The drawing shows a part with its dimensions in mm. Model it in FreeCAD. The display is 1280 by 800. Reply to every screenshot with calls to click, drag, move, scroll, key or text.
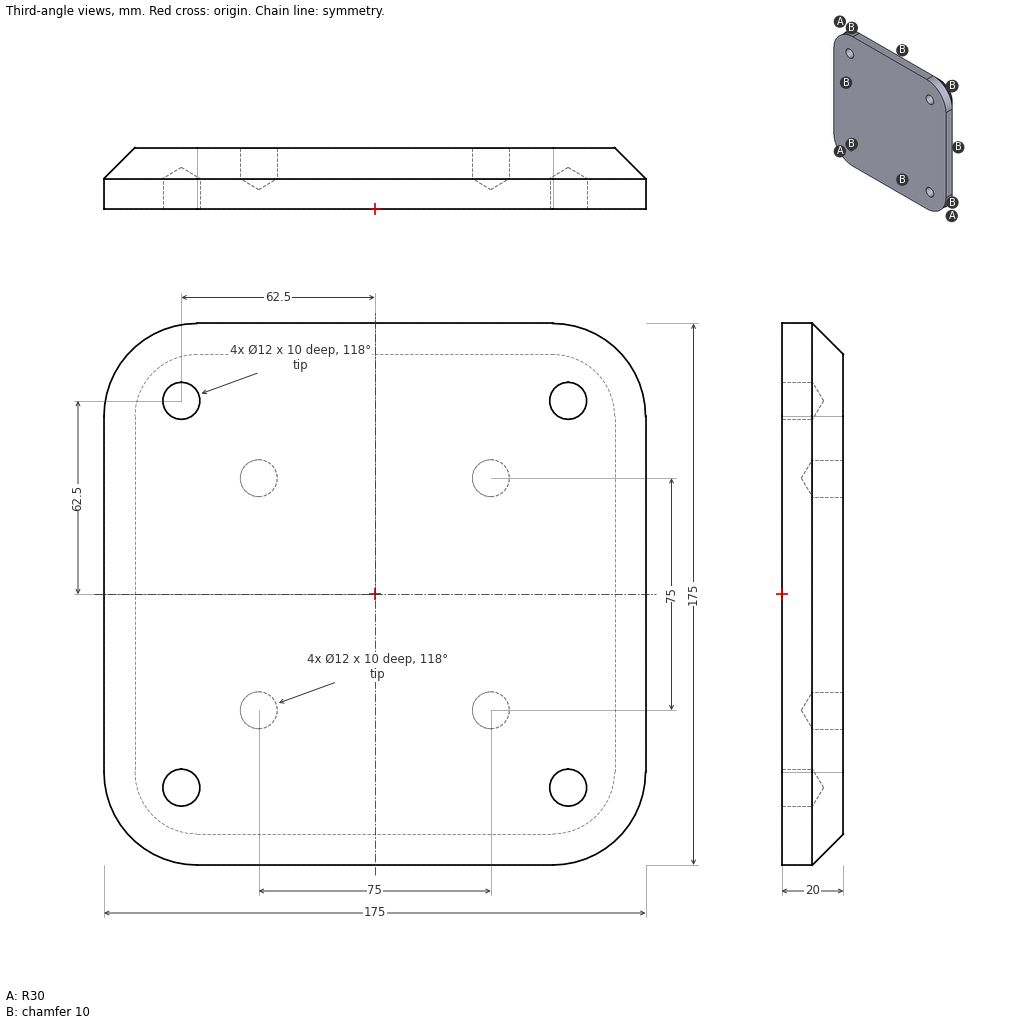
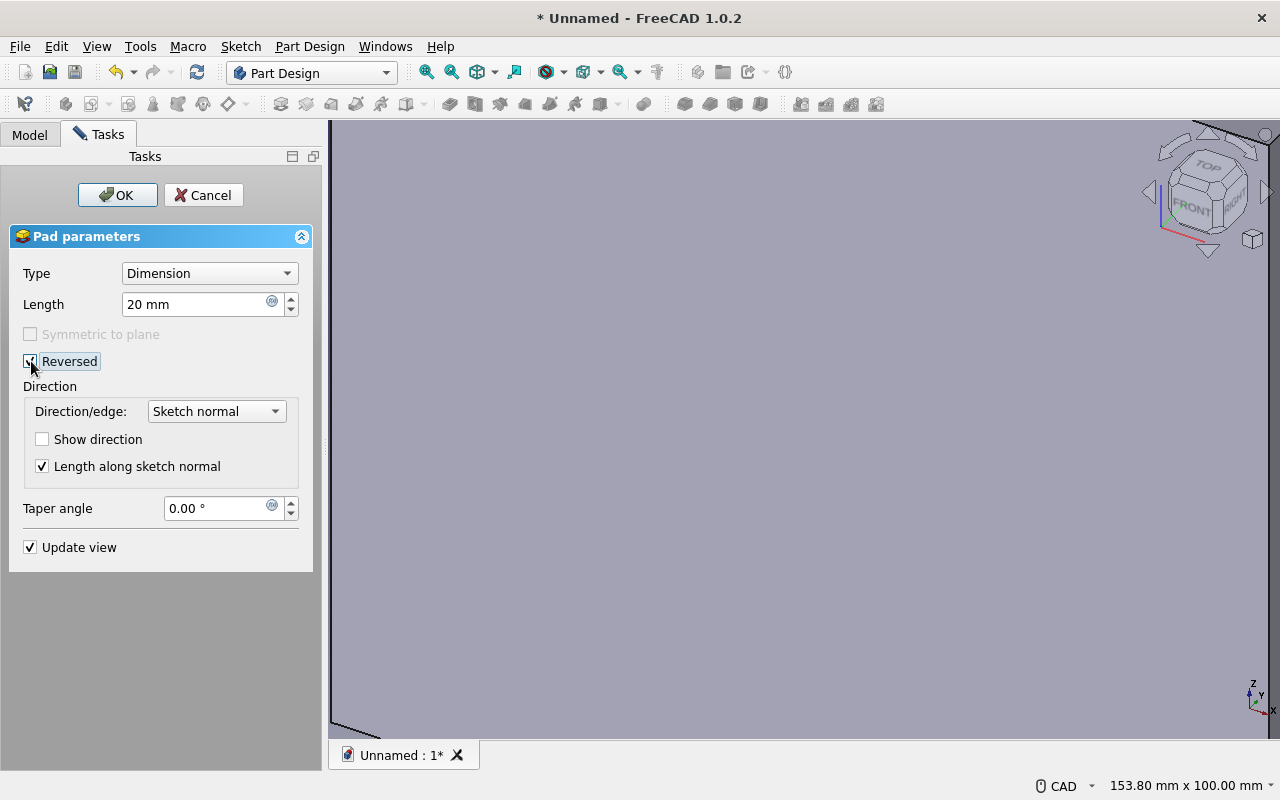
click(118, 195)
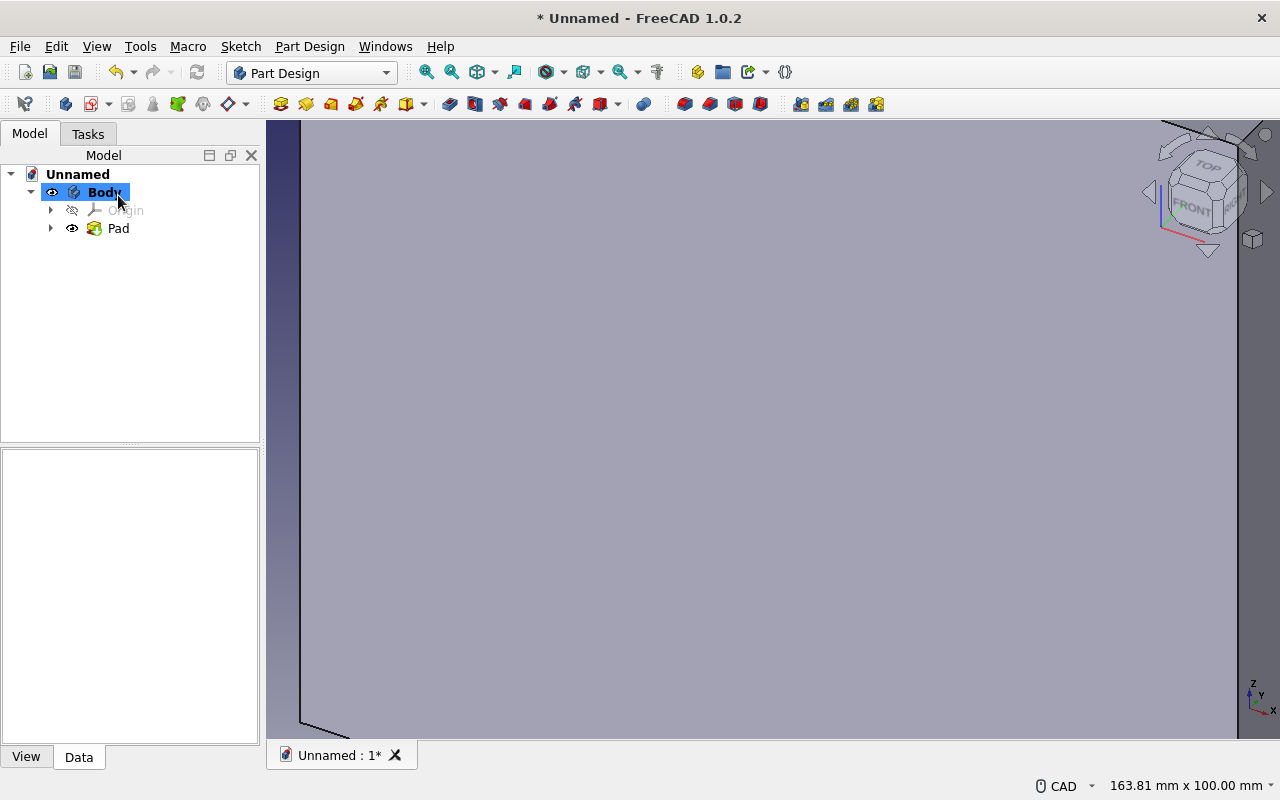
click(427, 72)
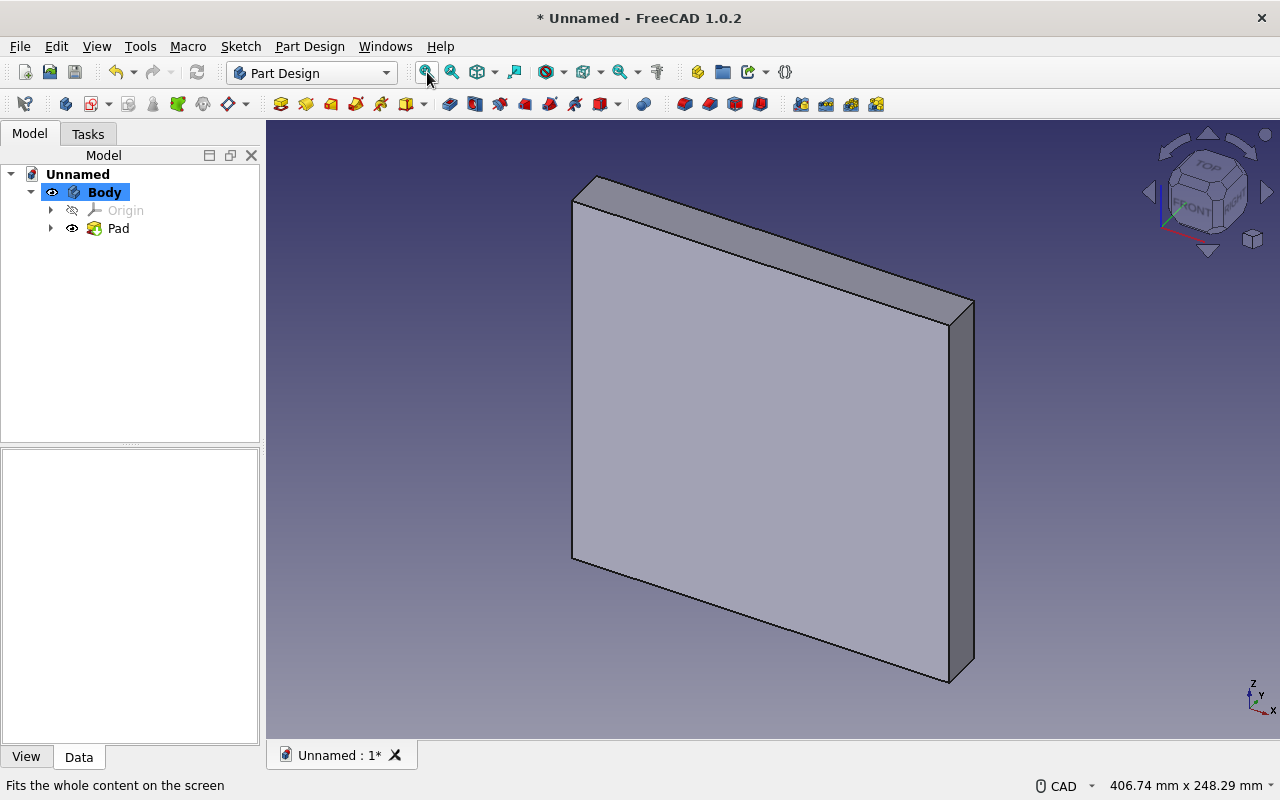
click(962, 312)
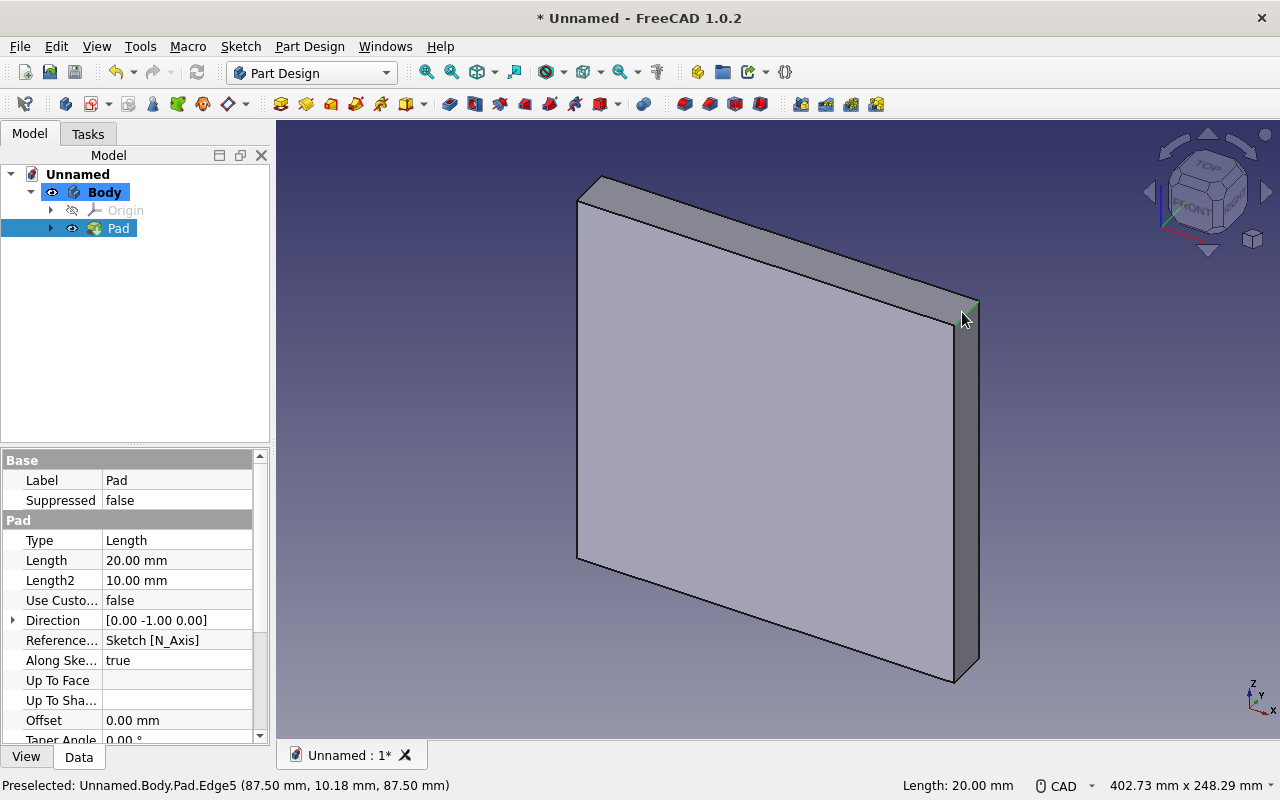
key(0)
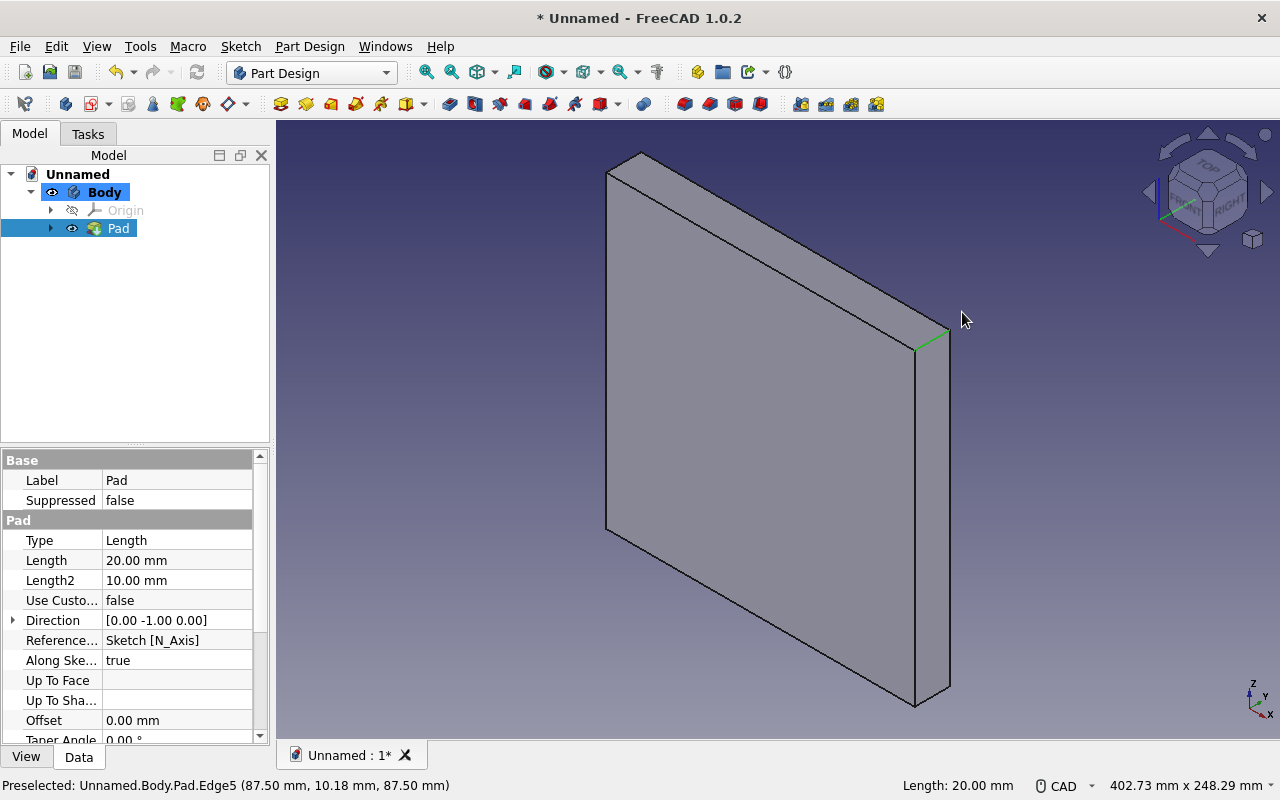
key(2)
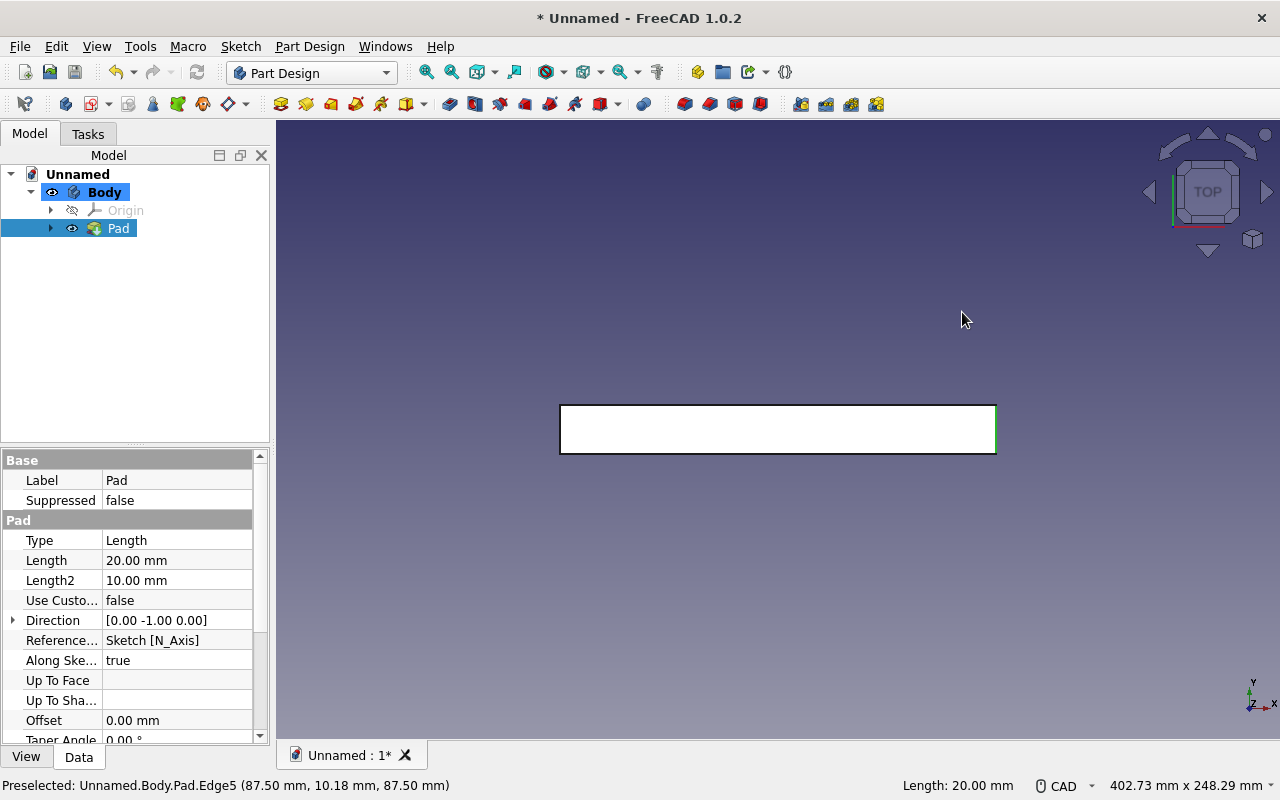
click(427, 72)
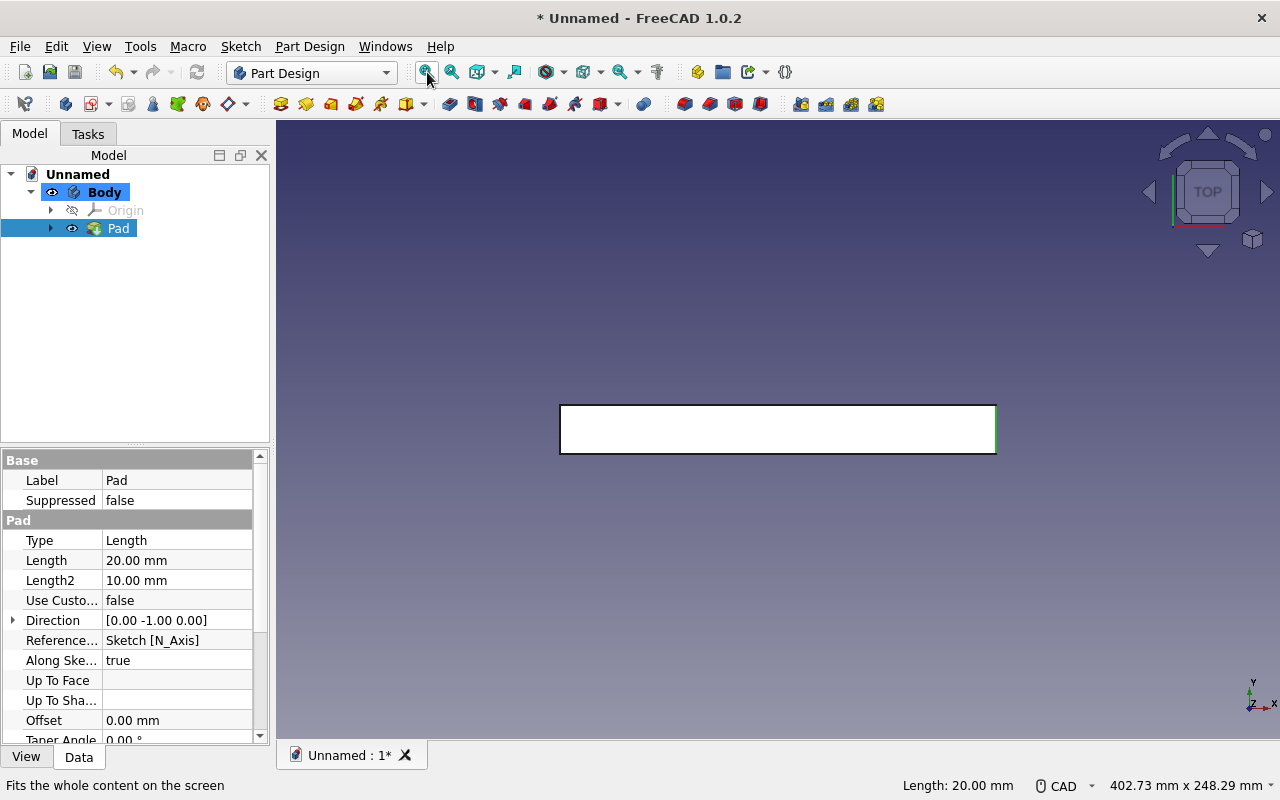
click(560, 428, ctrl)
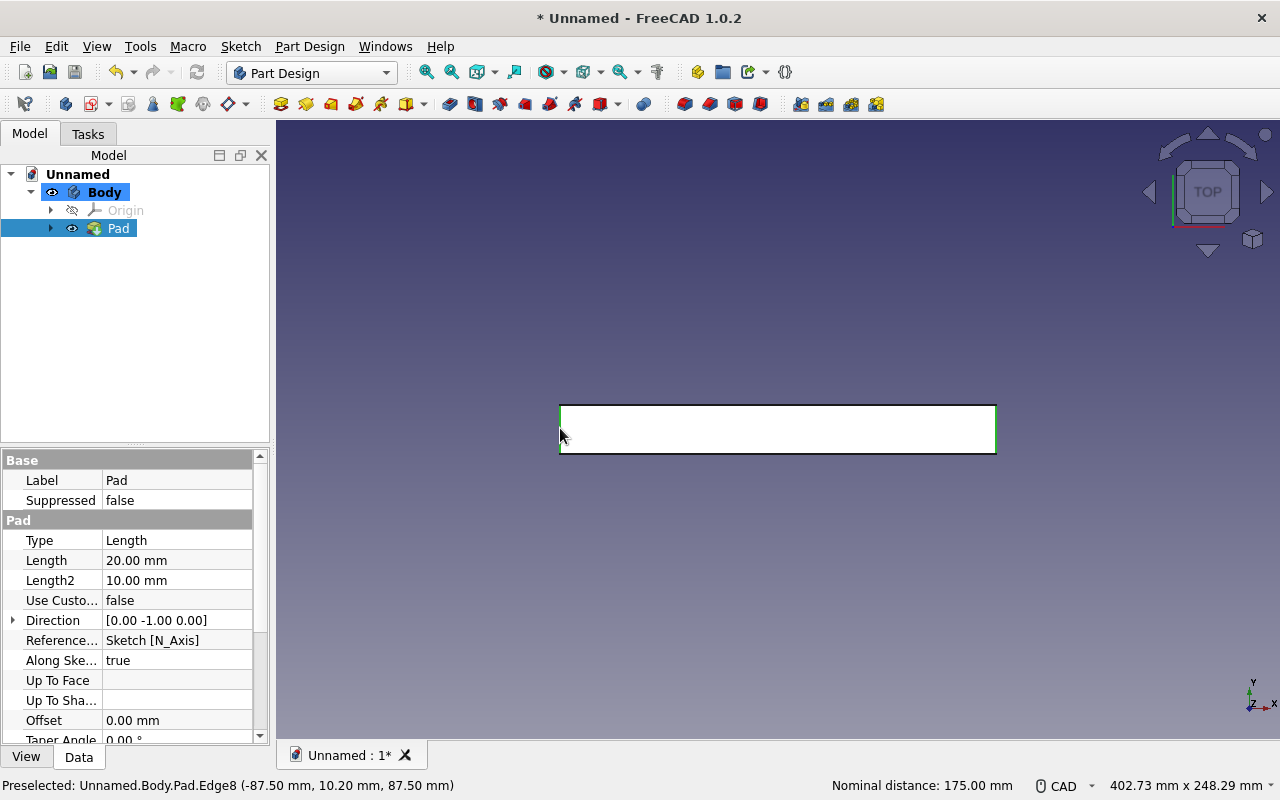
key(1)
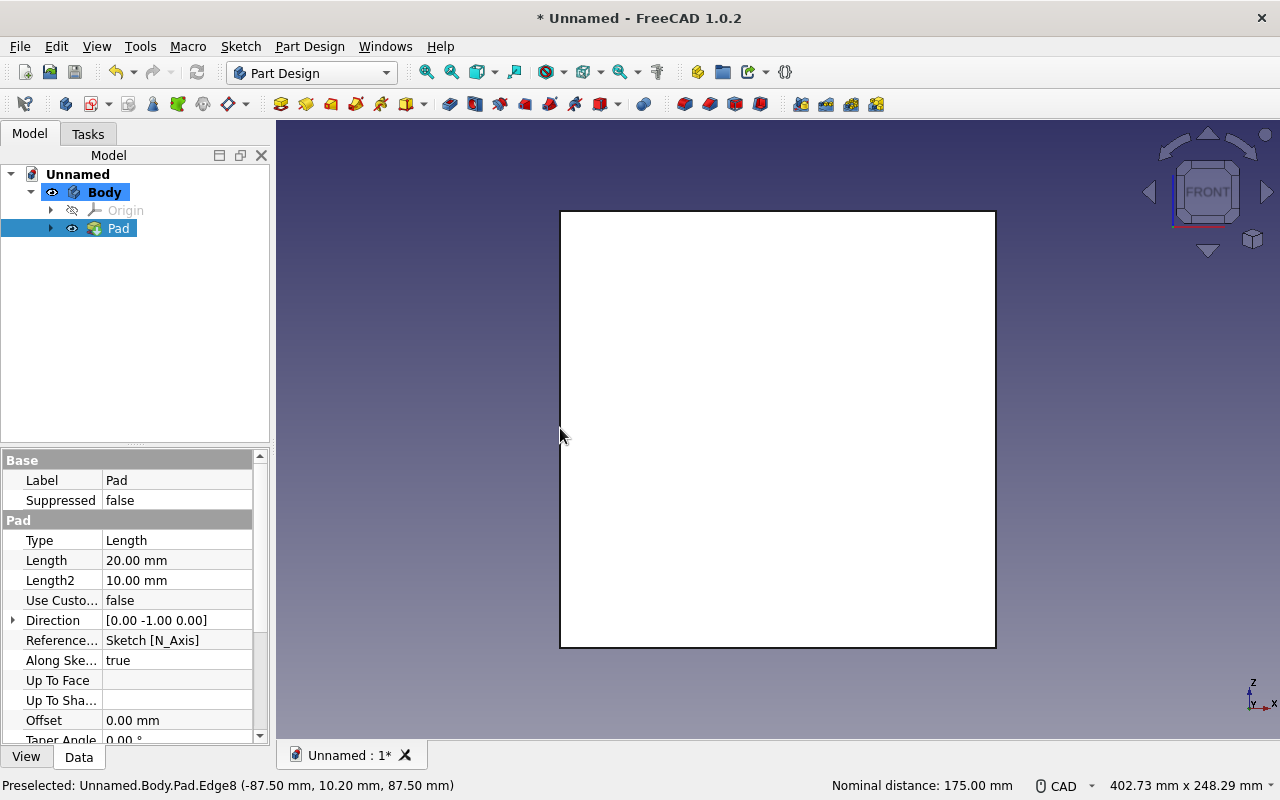
key(3)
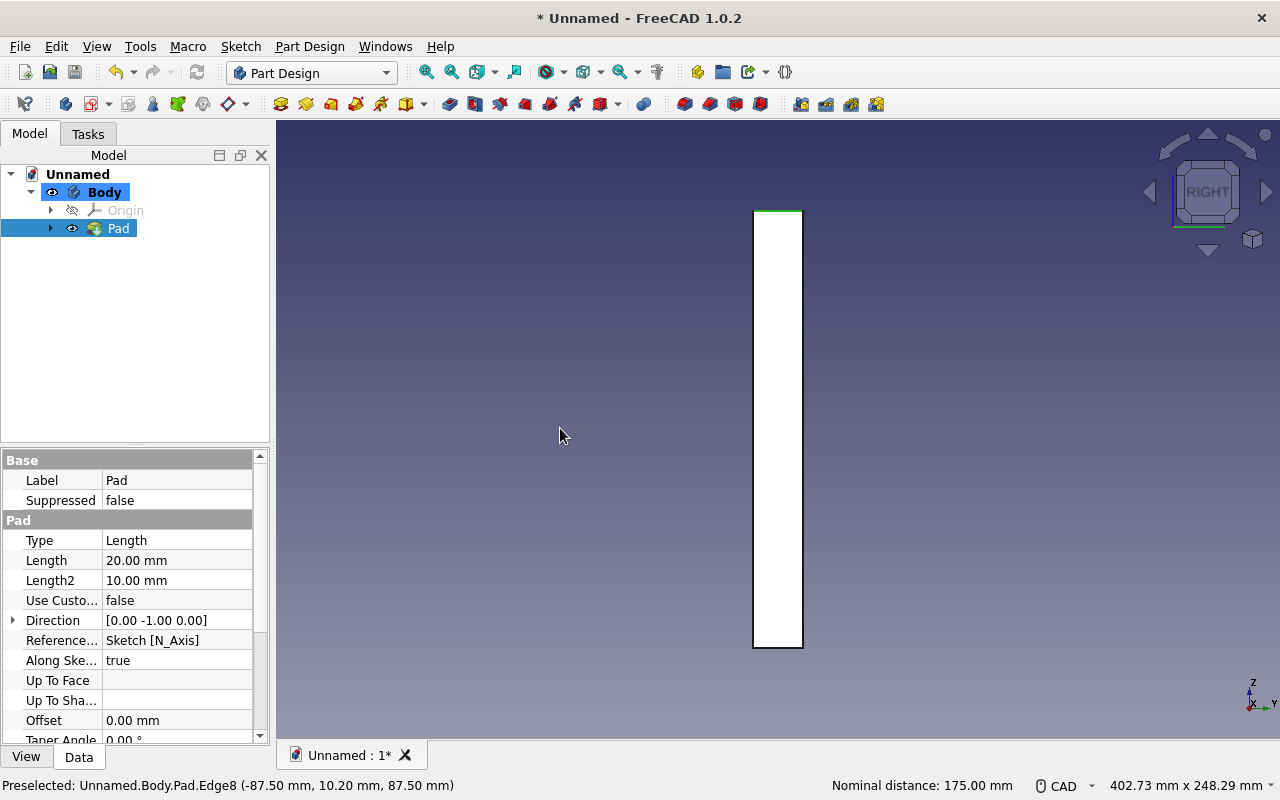
click(778, 647, ctrl)